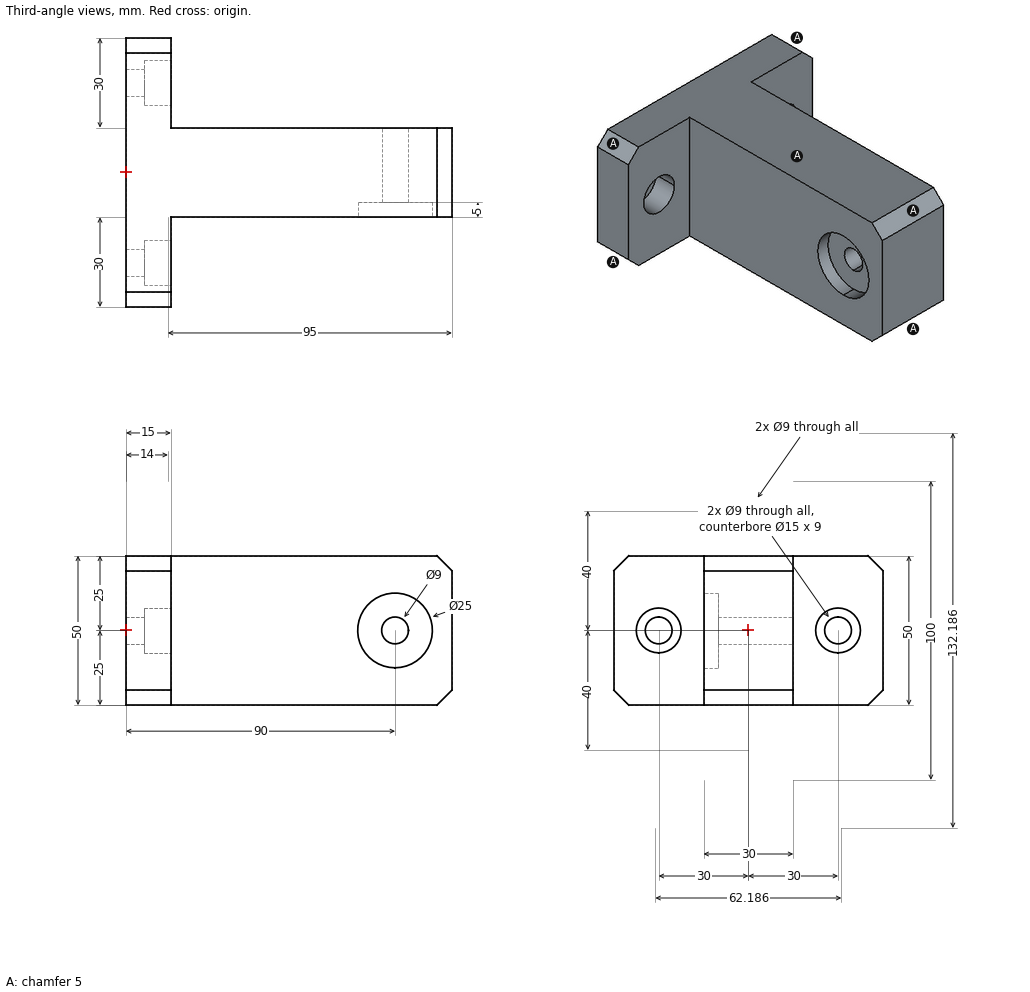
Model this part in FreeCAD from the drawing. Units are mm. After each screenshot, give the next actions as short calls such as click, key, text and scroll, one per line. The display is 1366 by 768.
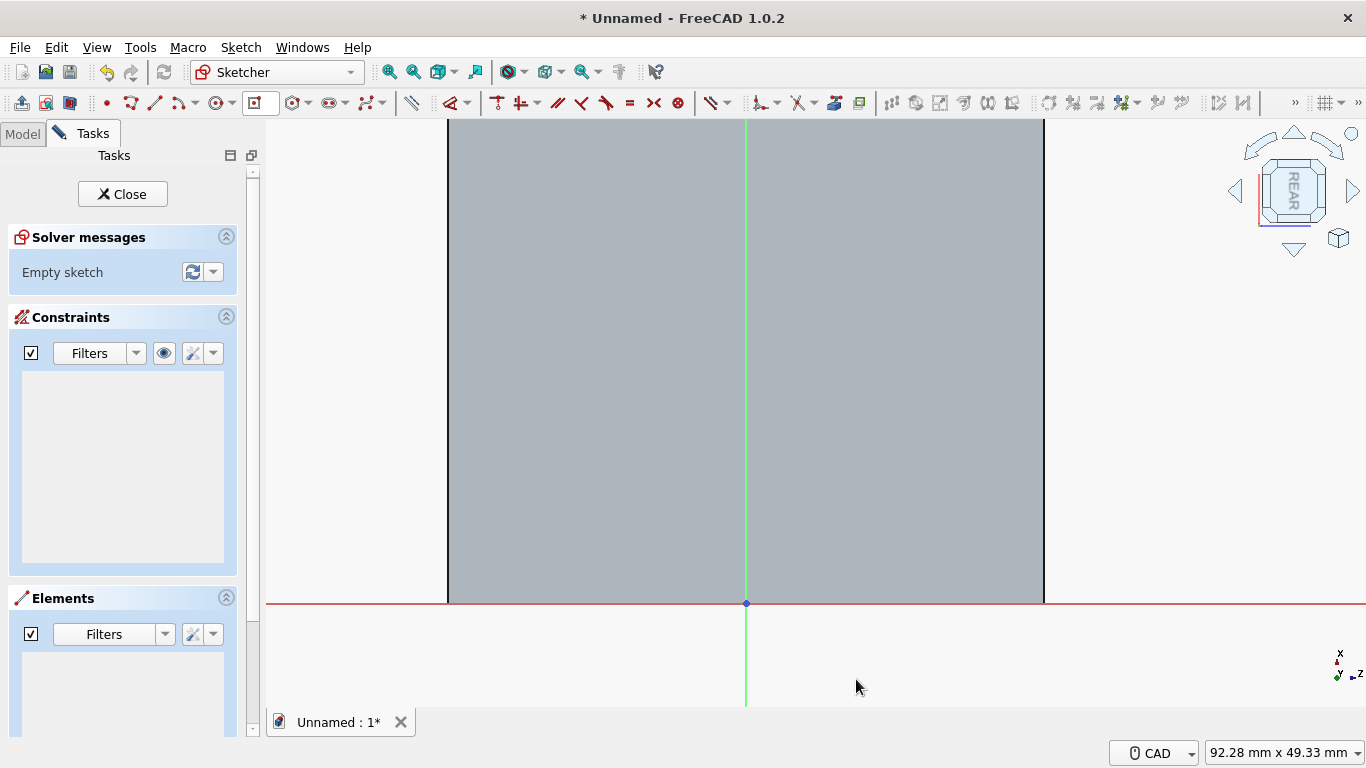
click(274, 104)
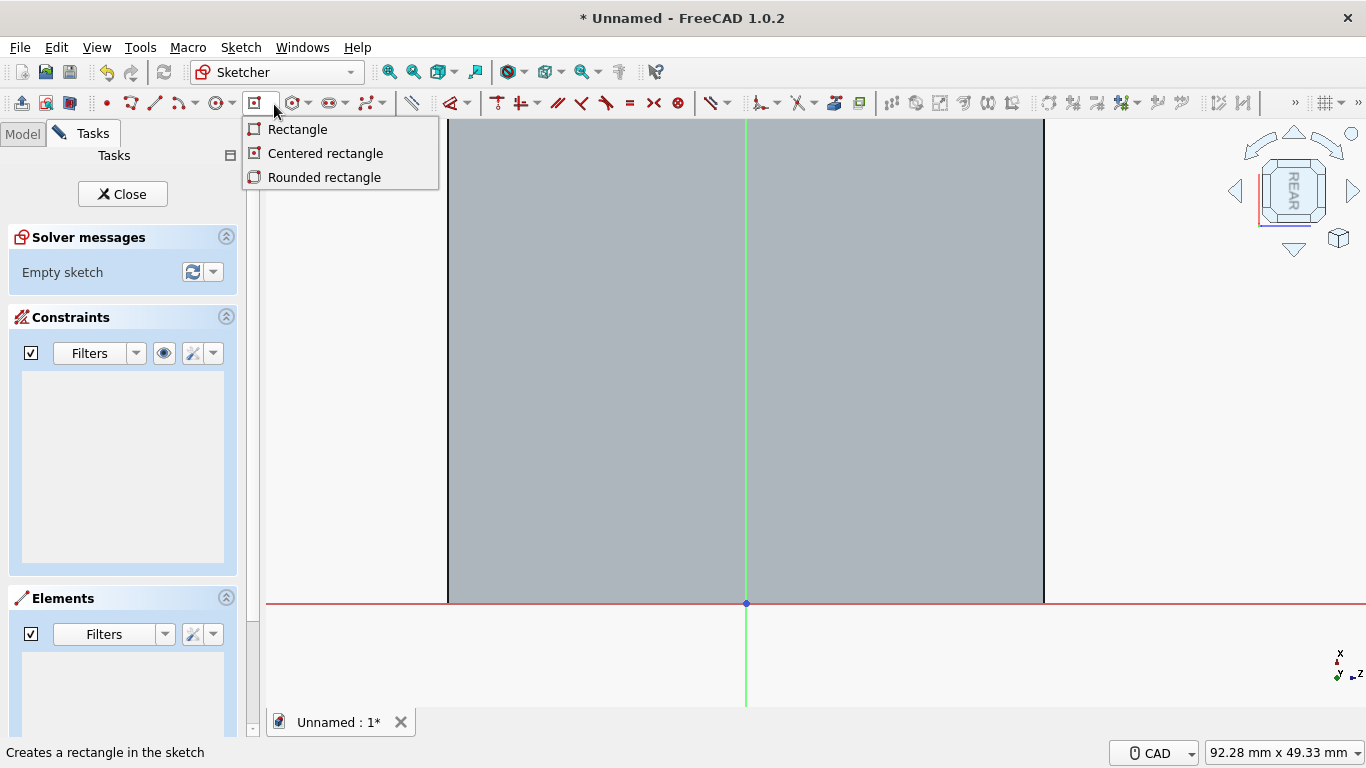
click(340, 129)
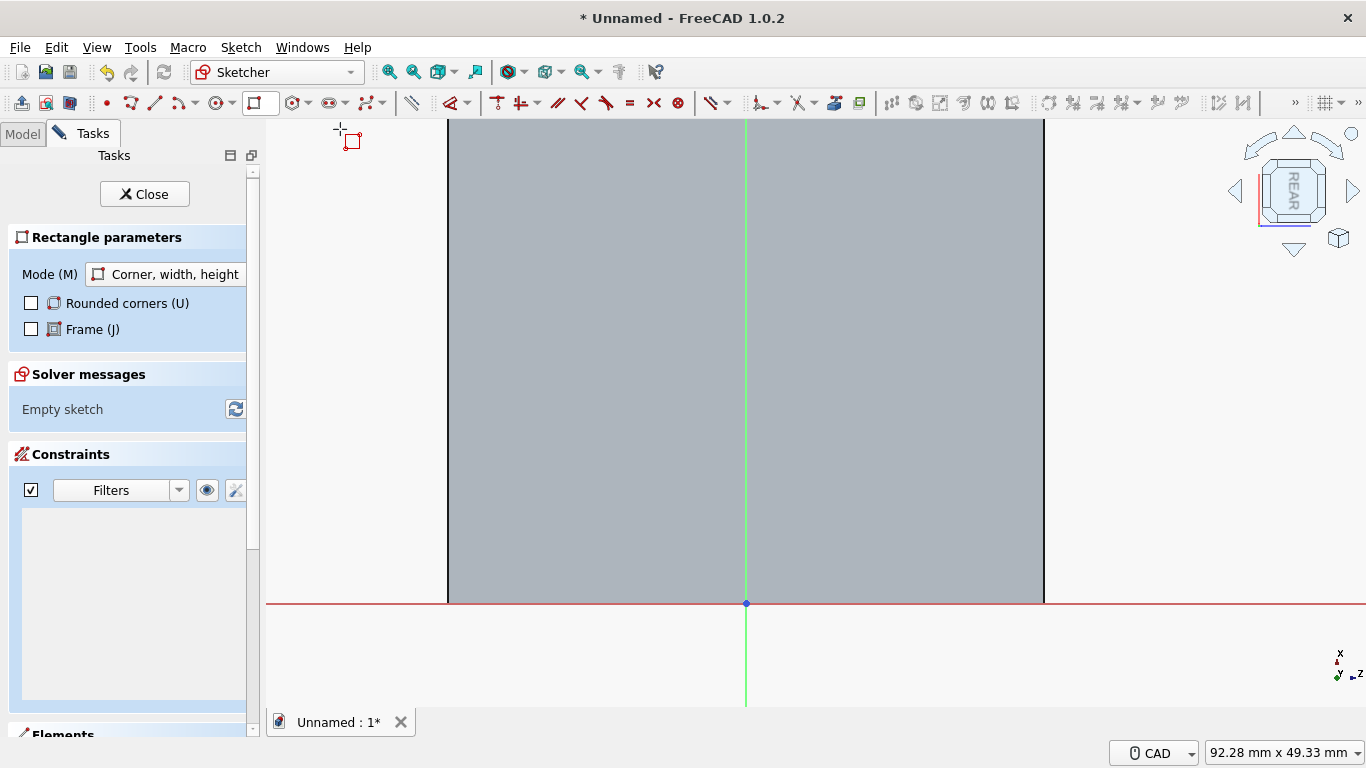
click(448, 425)
click(1044, 604)
key(Escape)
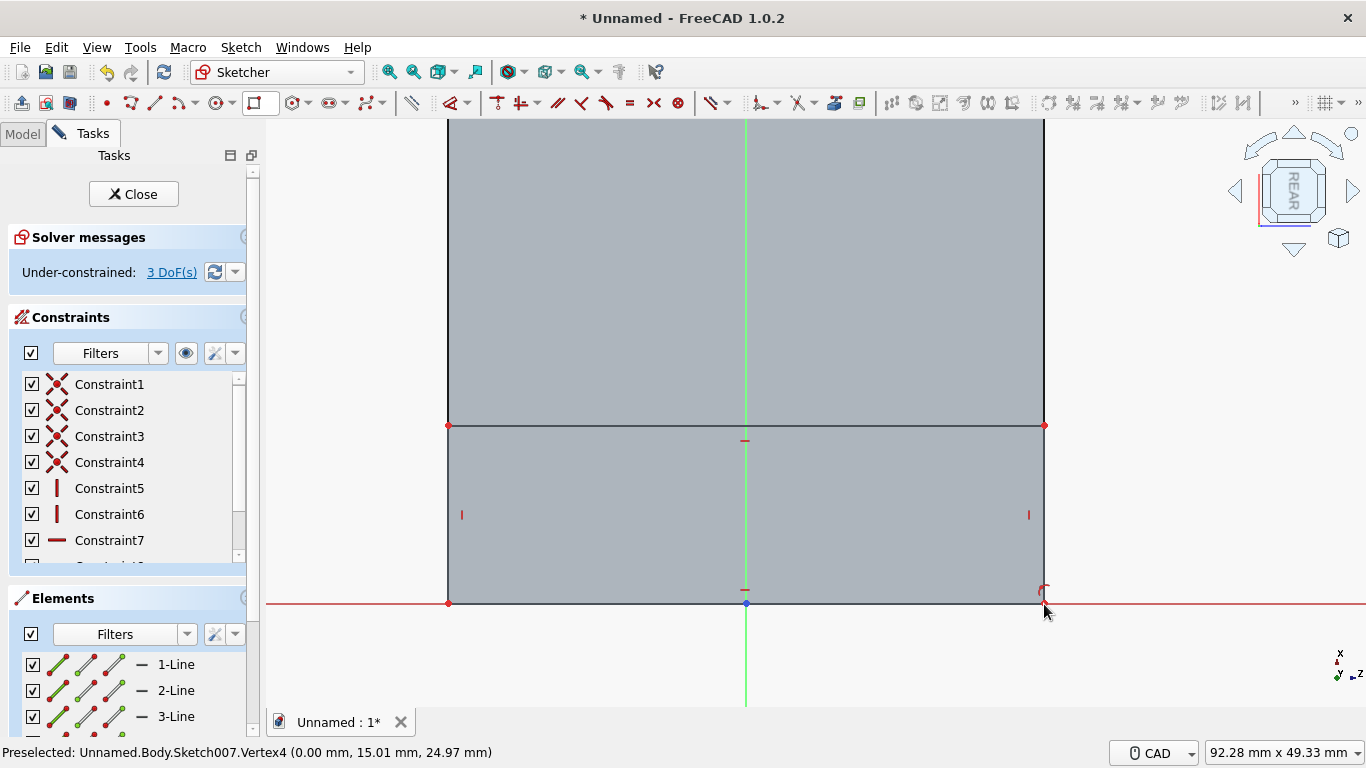
key(d)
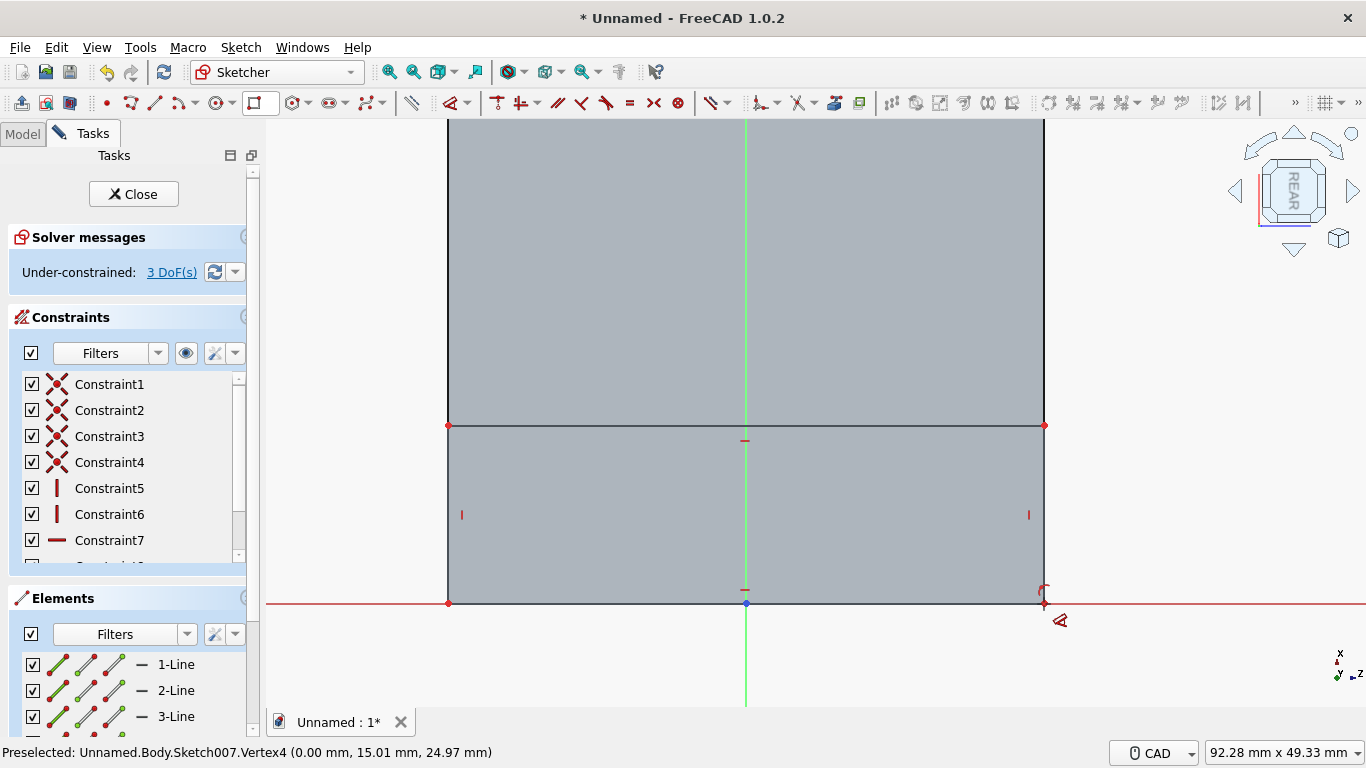
click(448, 479)
click(414, 515)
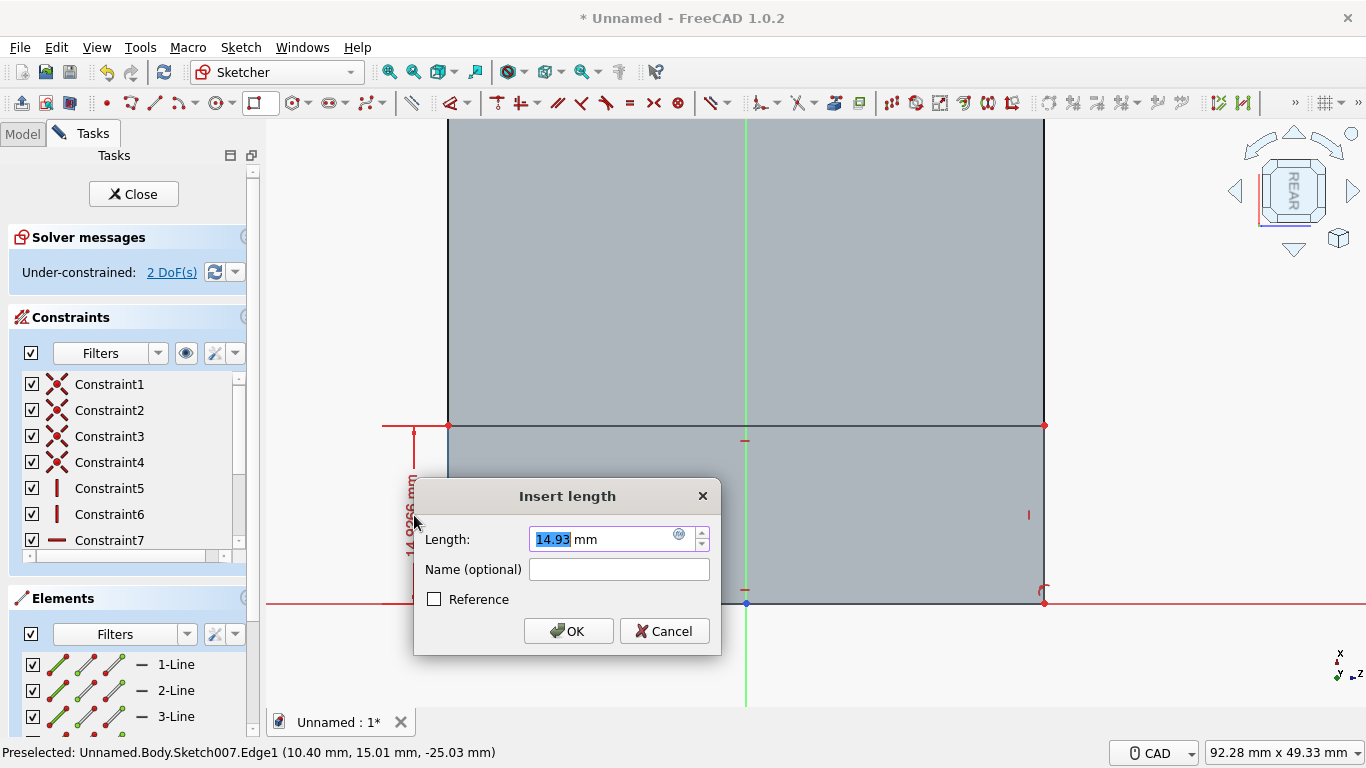
text(15)
key(Return)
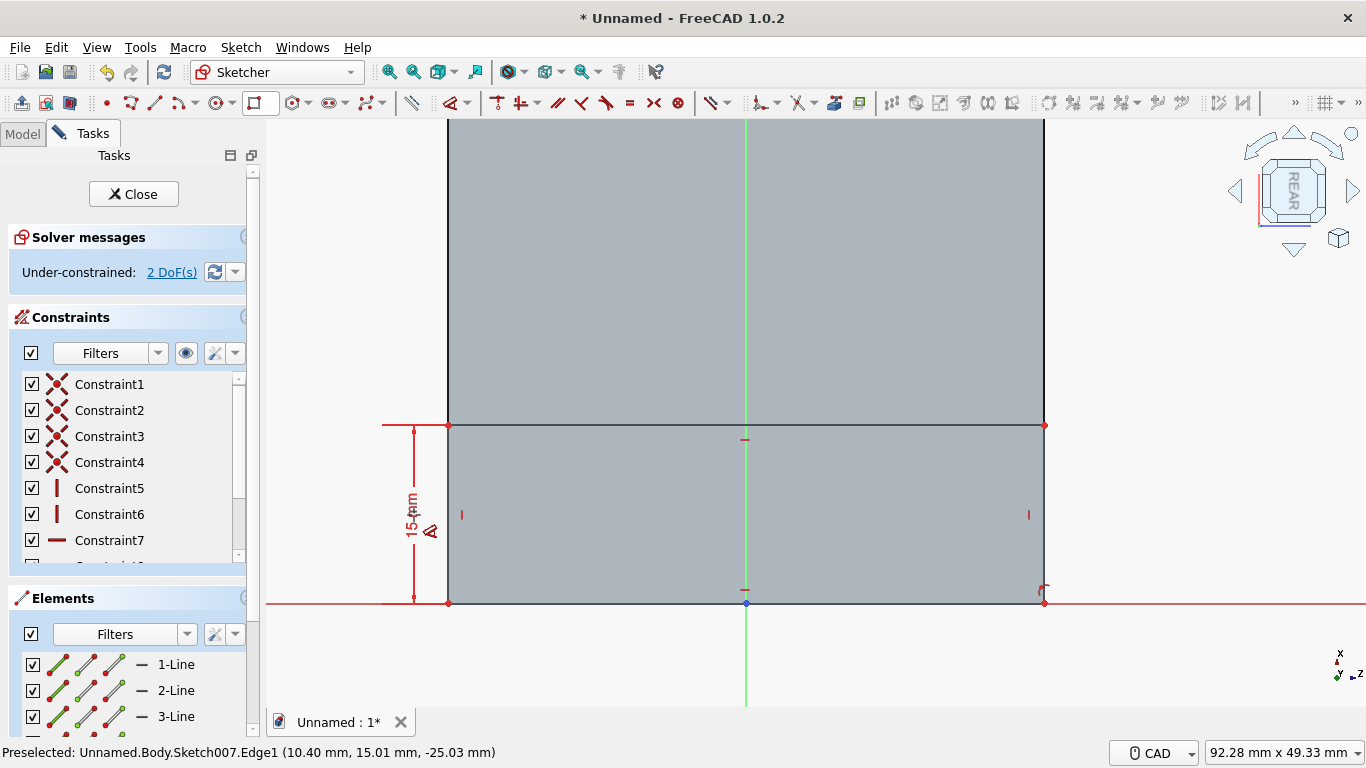
click(627, 604)
click(609, 638)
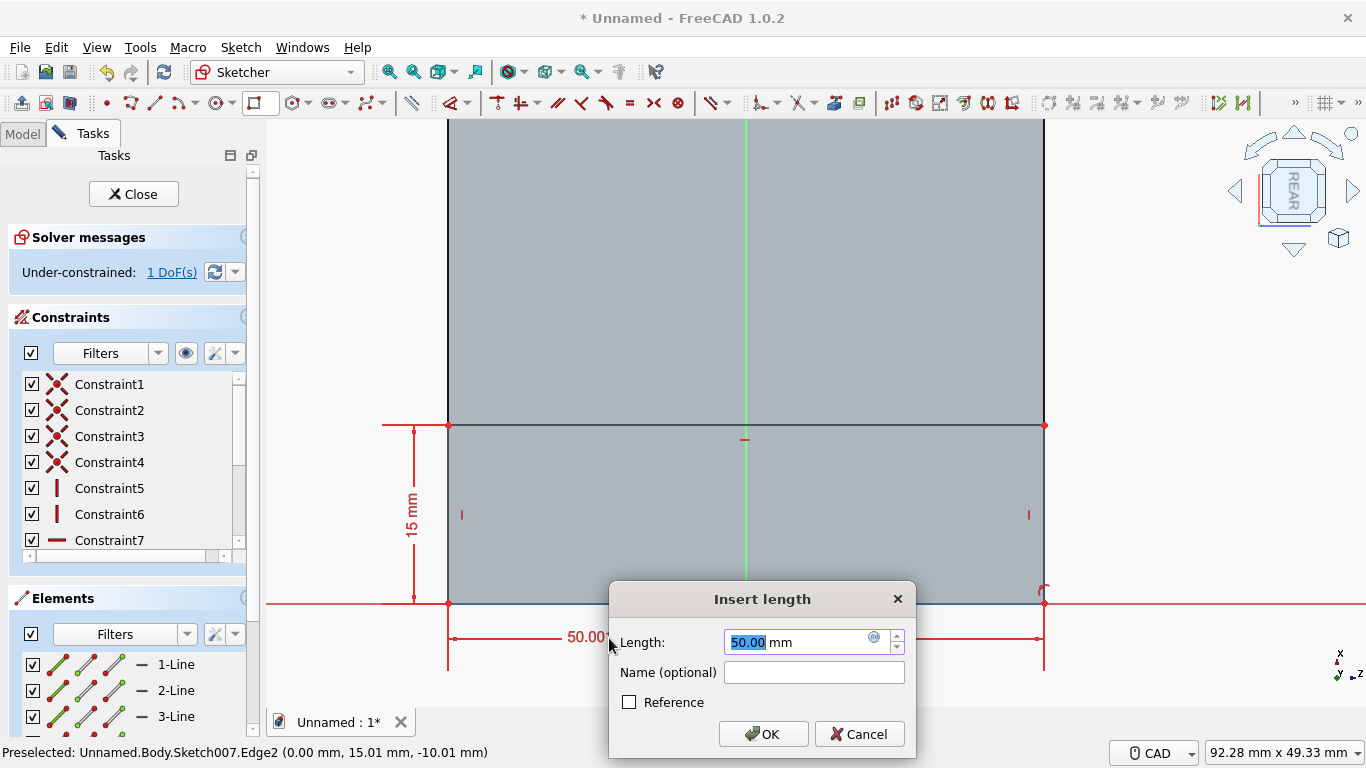
text(50)
key(Return)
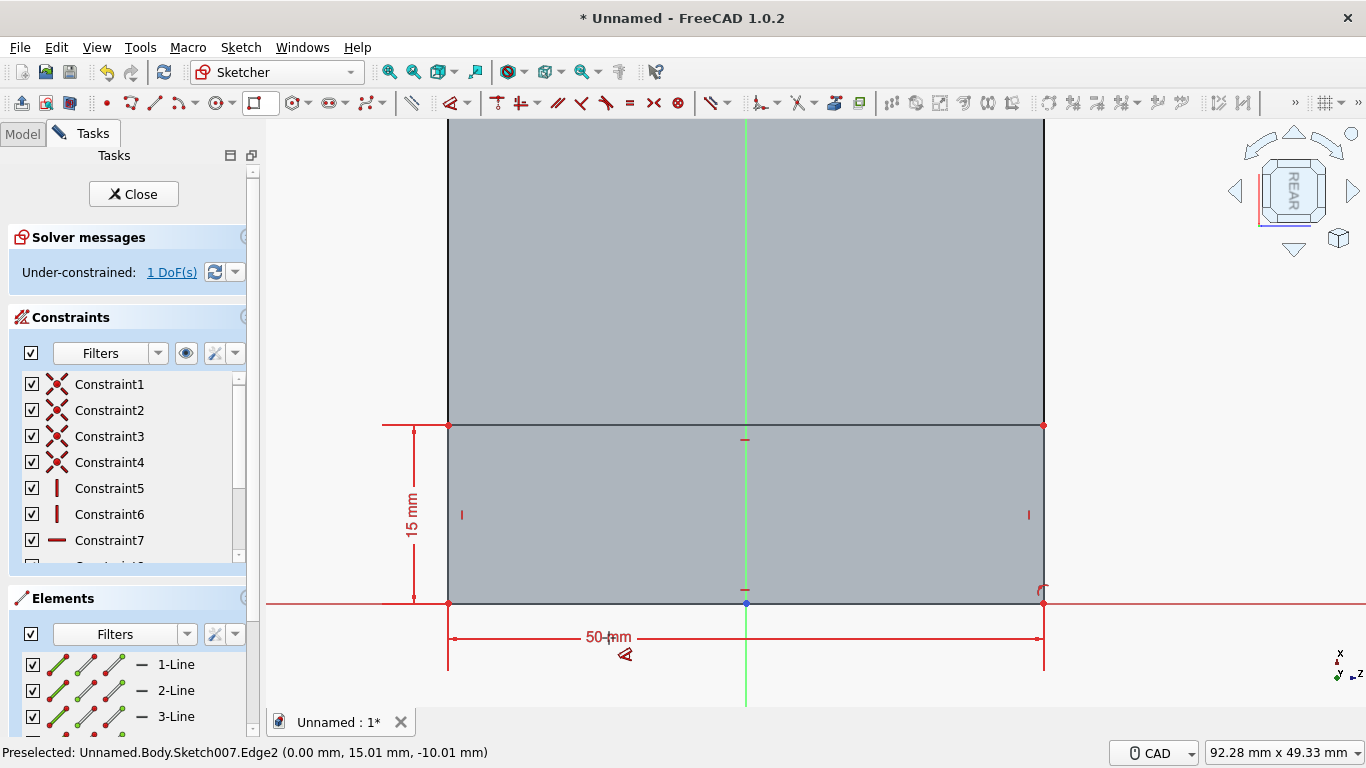
click(448, 425)
click(529, 638)